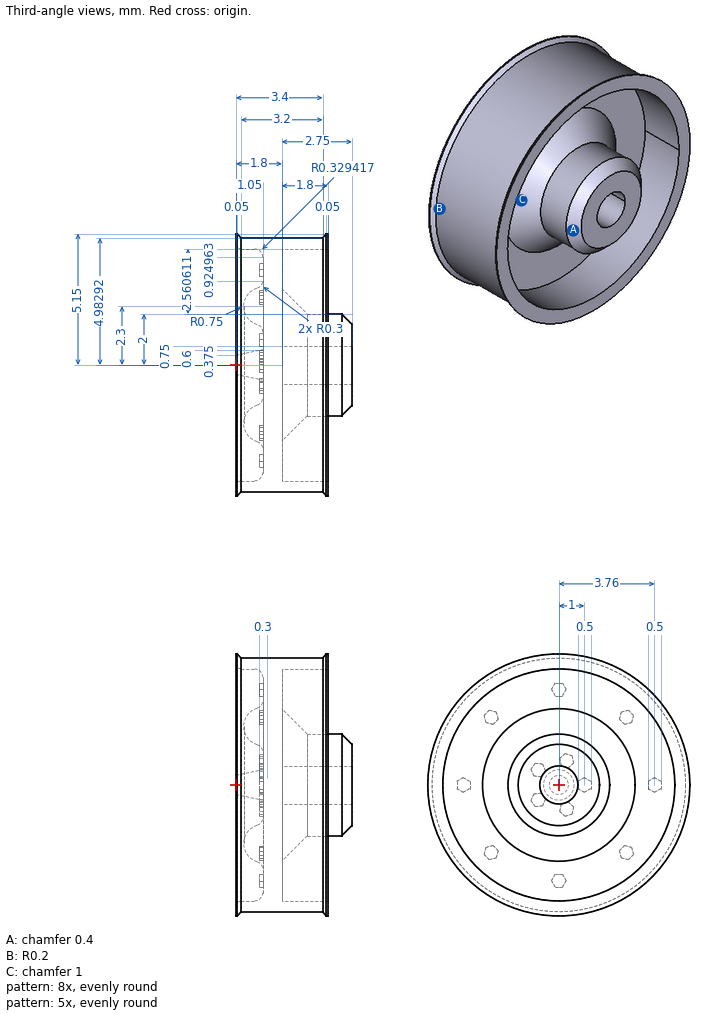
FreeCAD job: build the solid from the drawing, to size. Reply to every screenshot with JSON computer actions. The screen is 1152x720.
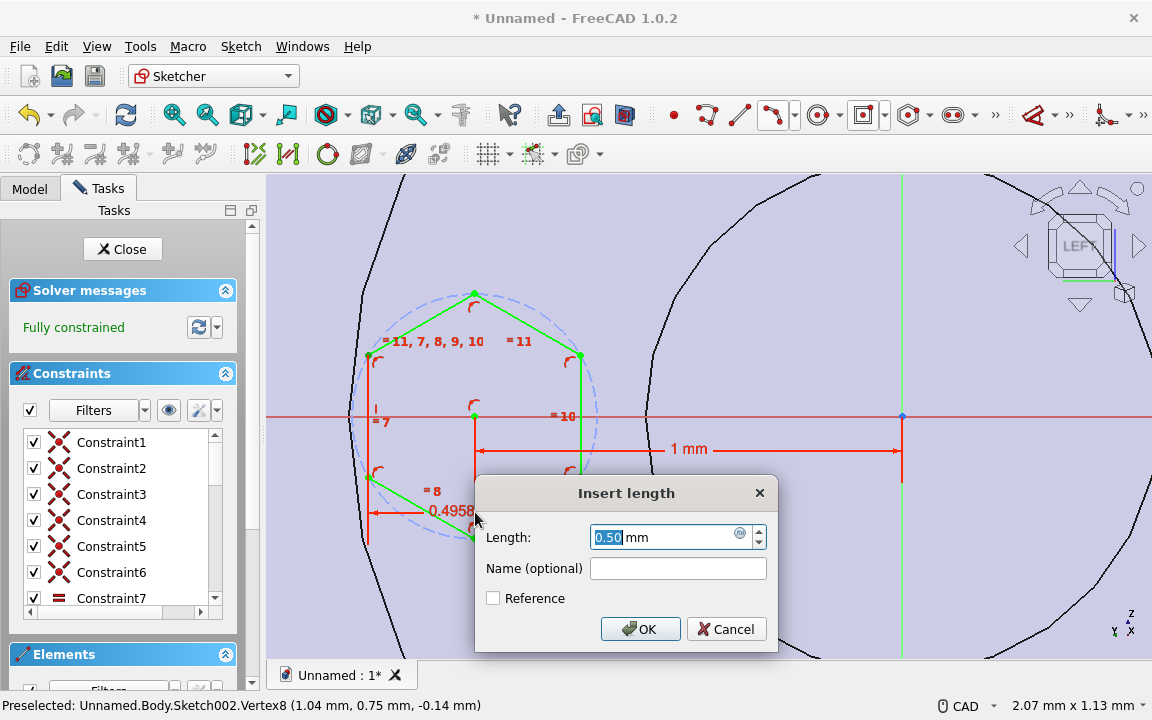
{"action": "type", "text": "0.5"}
{"action": "key", "text": "Return"}
{"action": "key", "text": "Escape"}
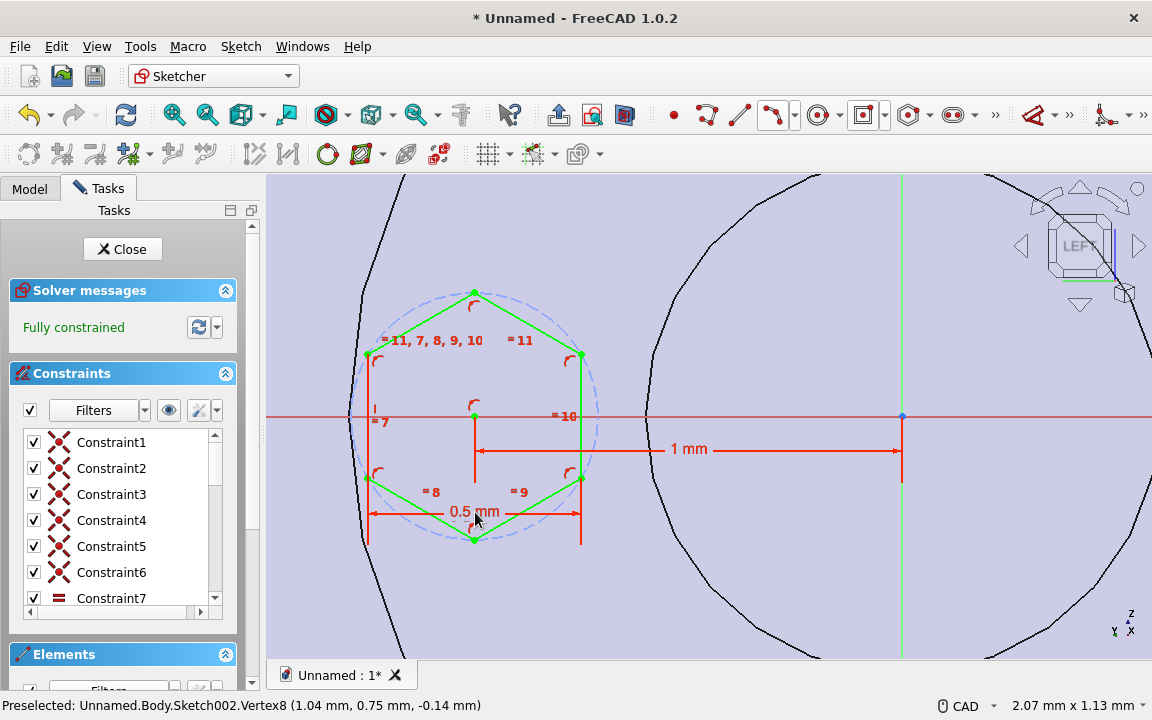
{"action": "left_click", "coordinate": [123, 249]}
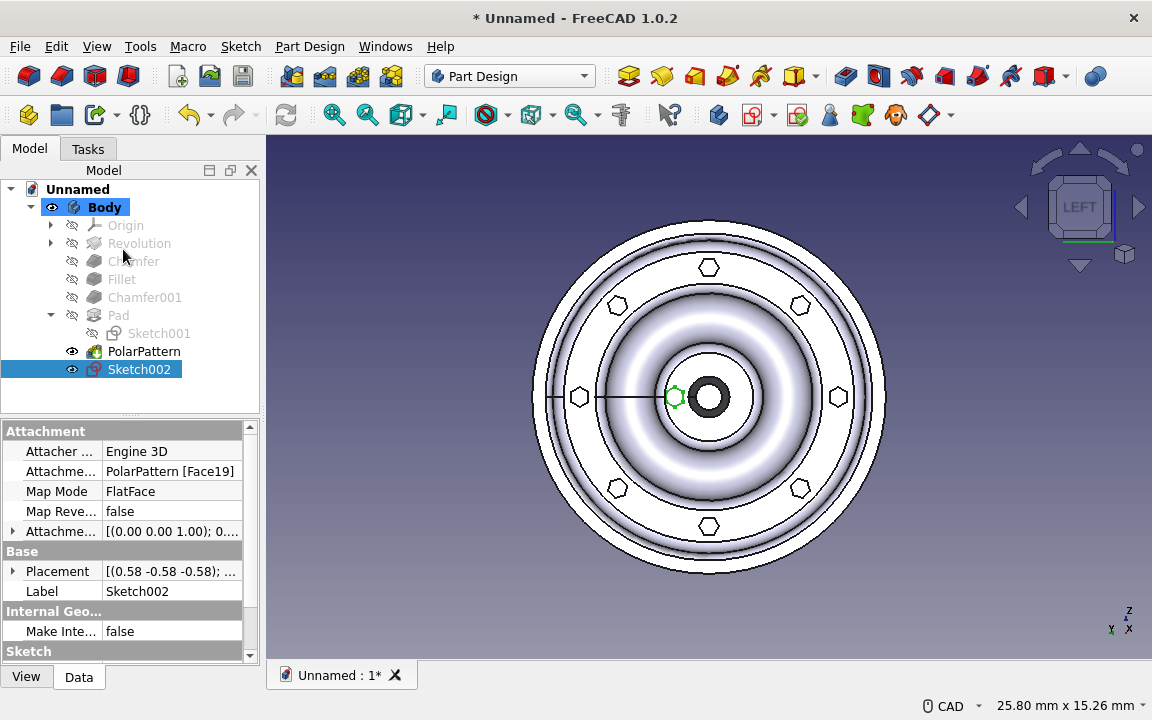
{"action": "left_click", "coordinate": [629, 76]}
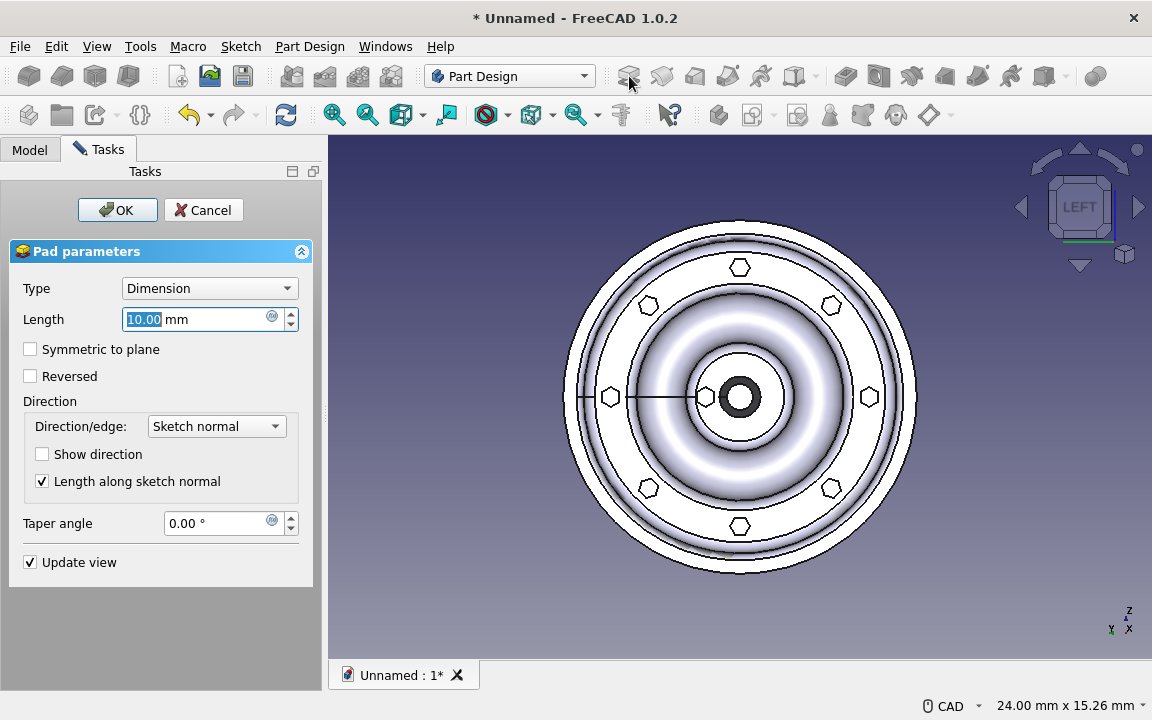
{"action": "type", "text": "0.3"}
{"action": "key", "text": "Tab"}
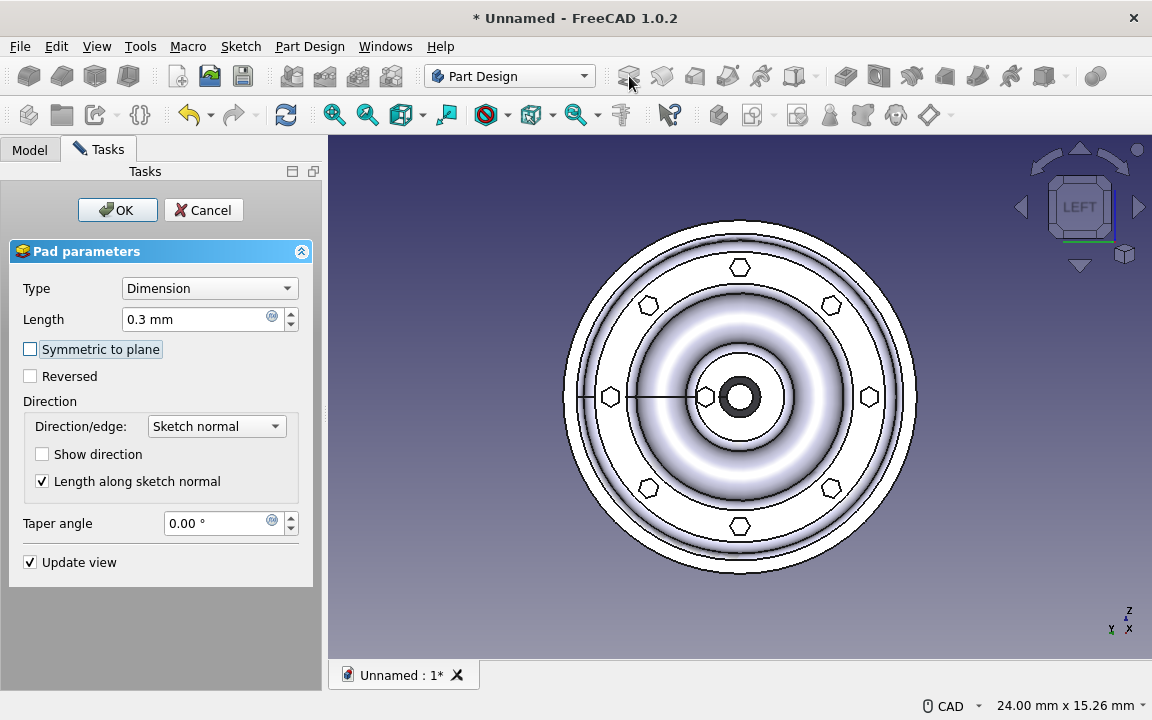
{"action": "left_click", "coordinate": [31, 349]}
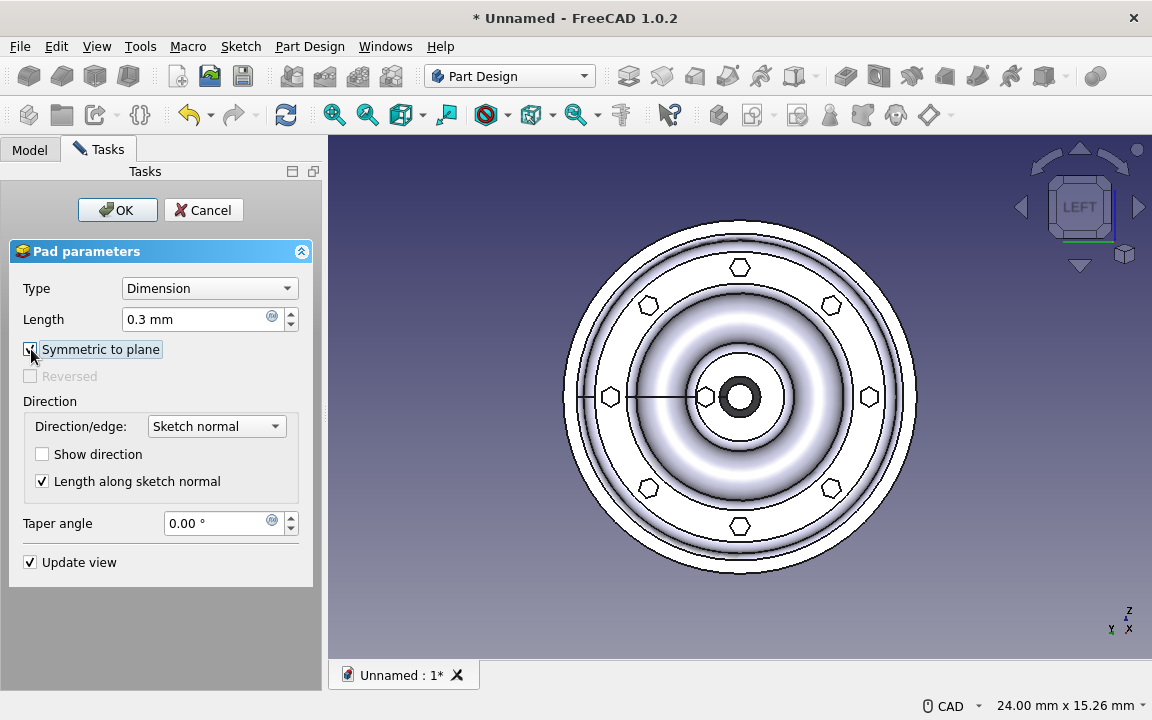
{"action": "left_click", "coordinate": [118, 210]}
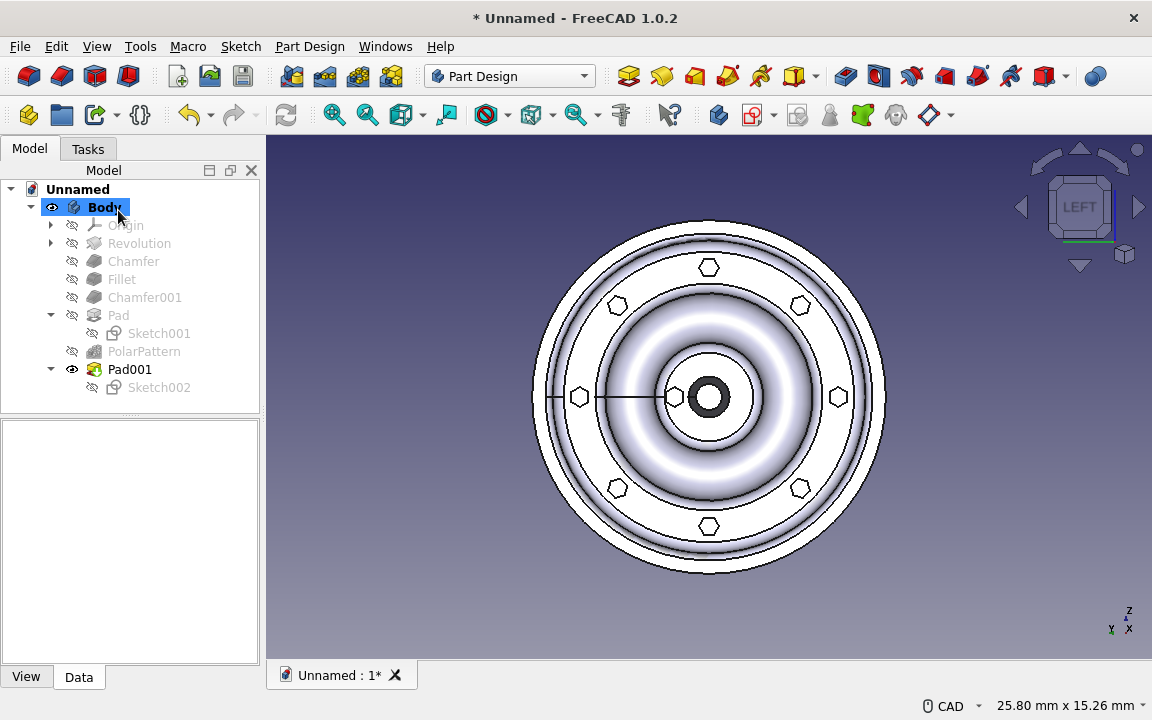
{"action": "left_click", "coordinate": [117, 369]}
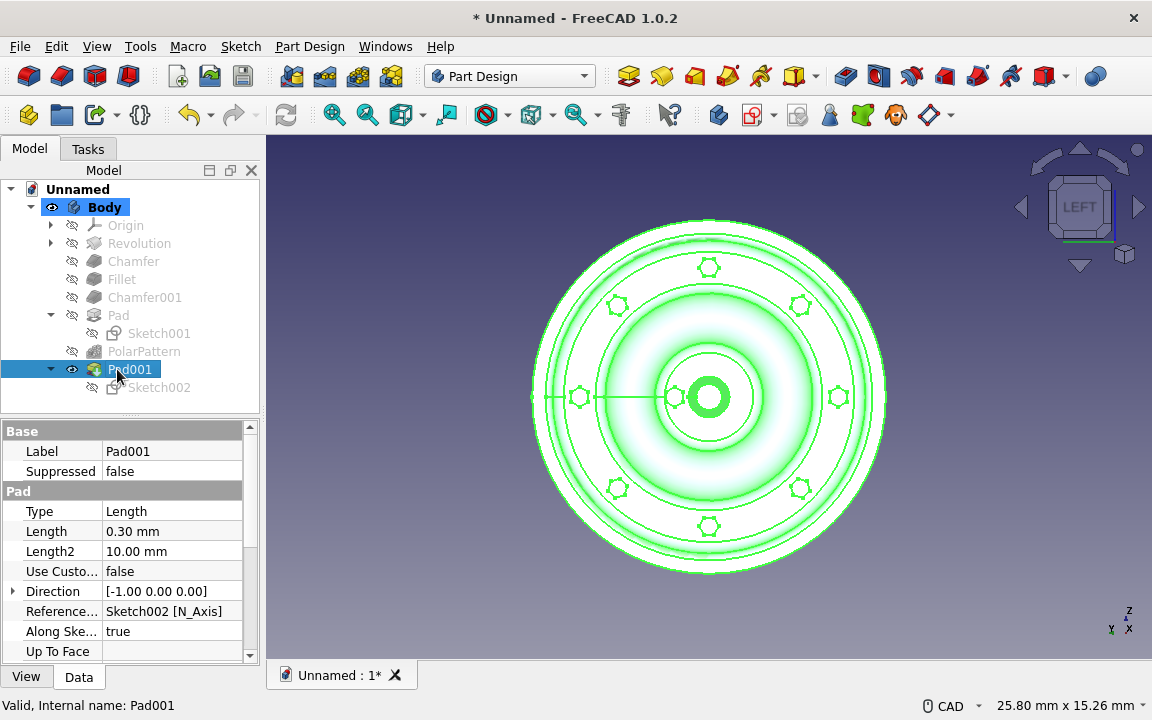
{"action": "left_click", "coordinate": [358, 76]}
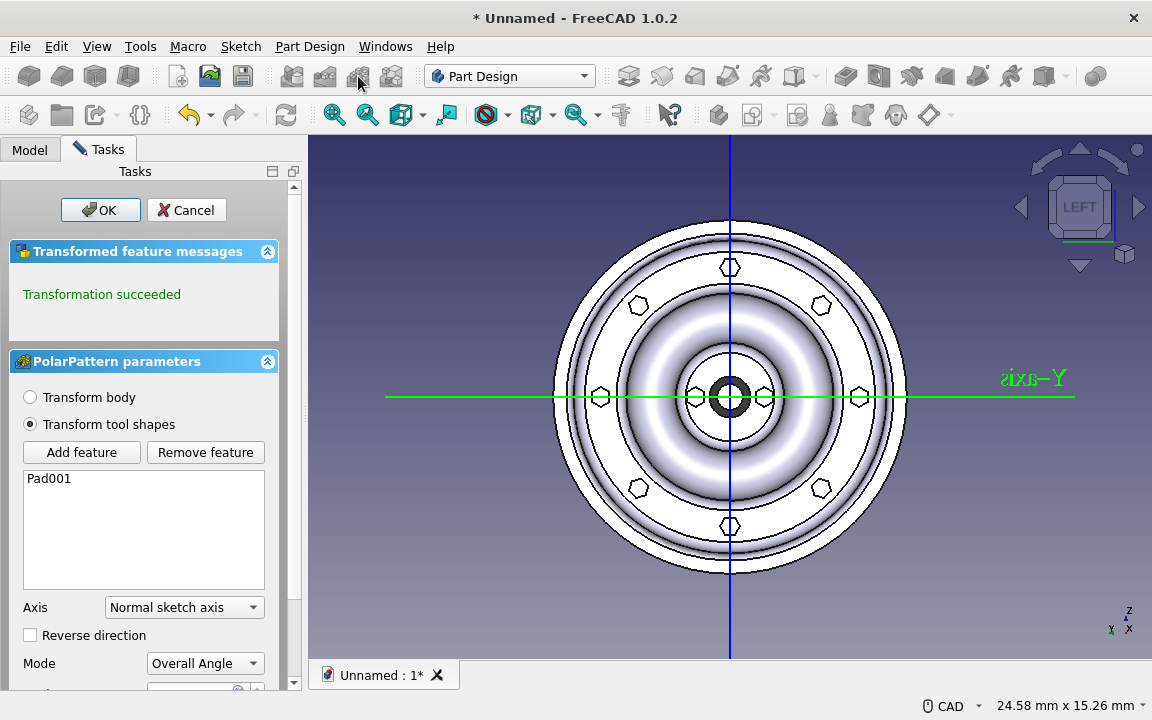
{"action": "left_click", "coordinate": [185, 608]}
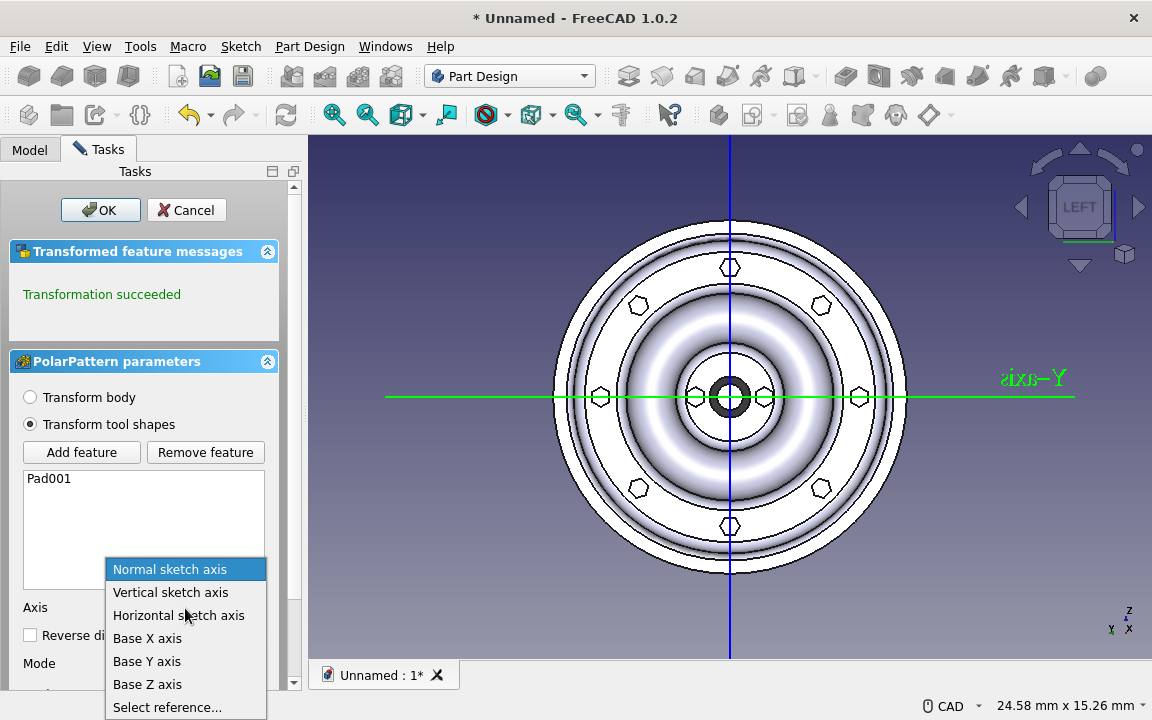
{"action": "left_click", "coordinate": [184, 638]}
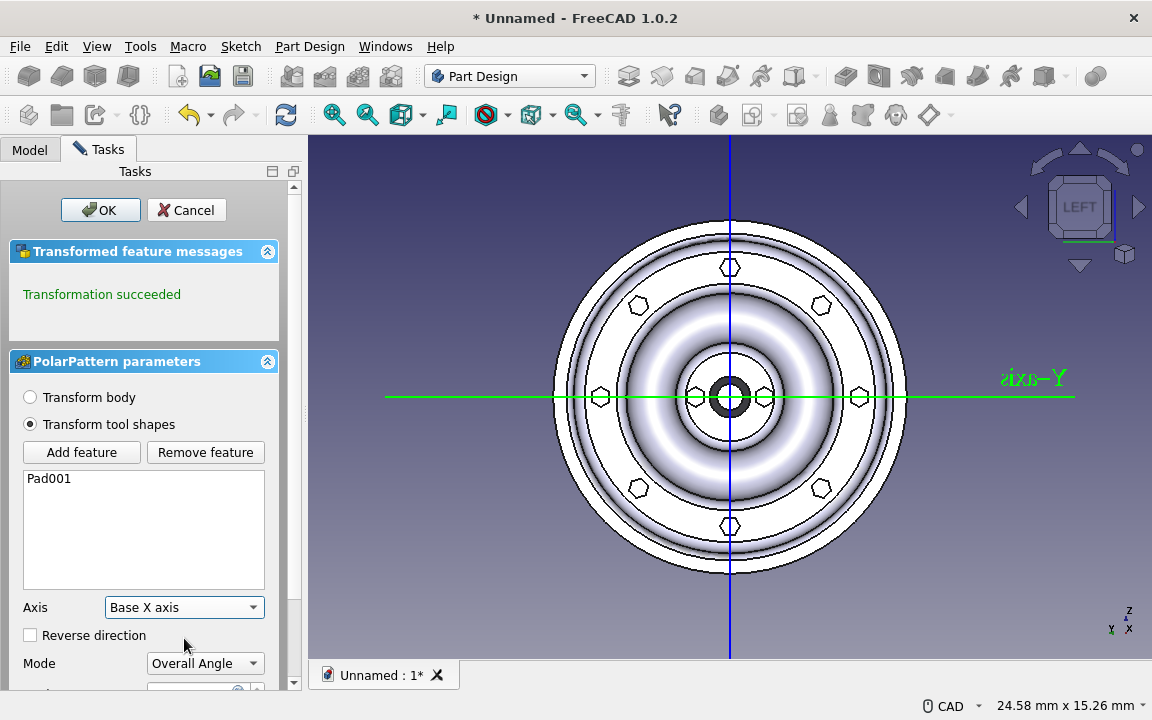
{"action": "scroll", "coordinate": [294, 436], "scroll_direction": "down", "scroll_amount": 2}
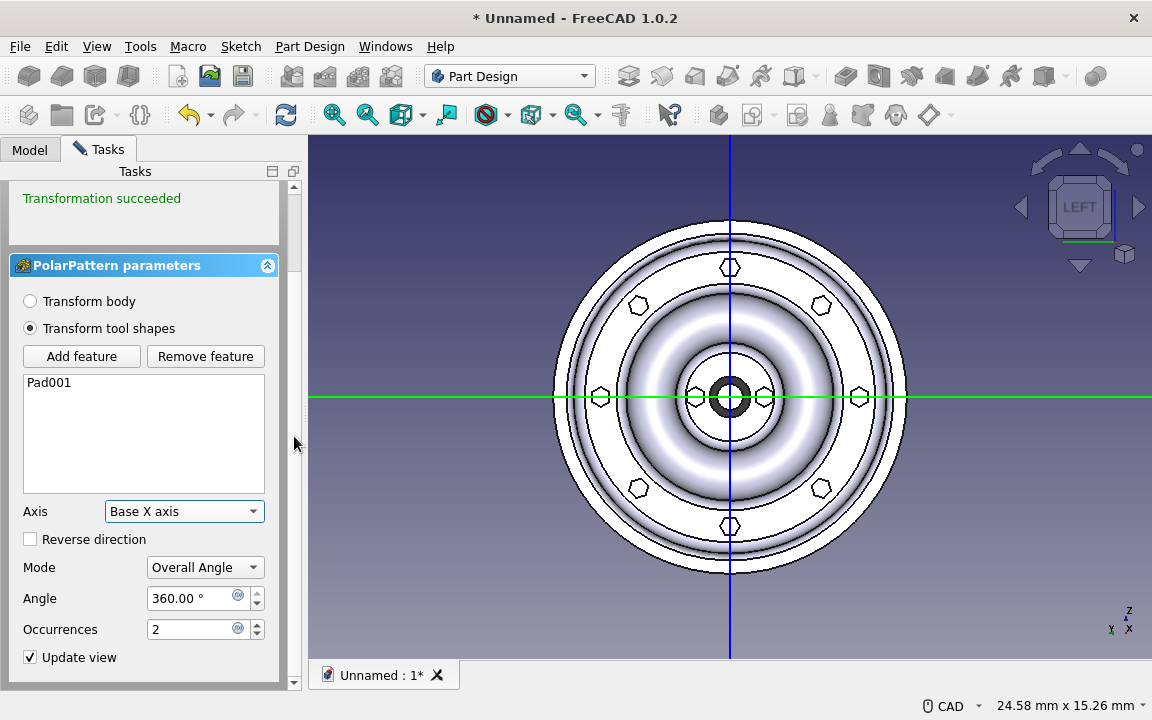
{"action": "triple_click", "coordinate": [199, 630]}